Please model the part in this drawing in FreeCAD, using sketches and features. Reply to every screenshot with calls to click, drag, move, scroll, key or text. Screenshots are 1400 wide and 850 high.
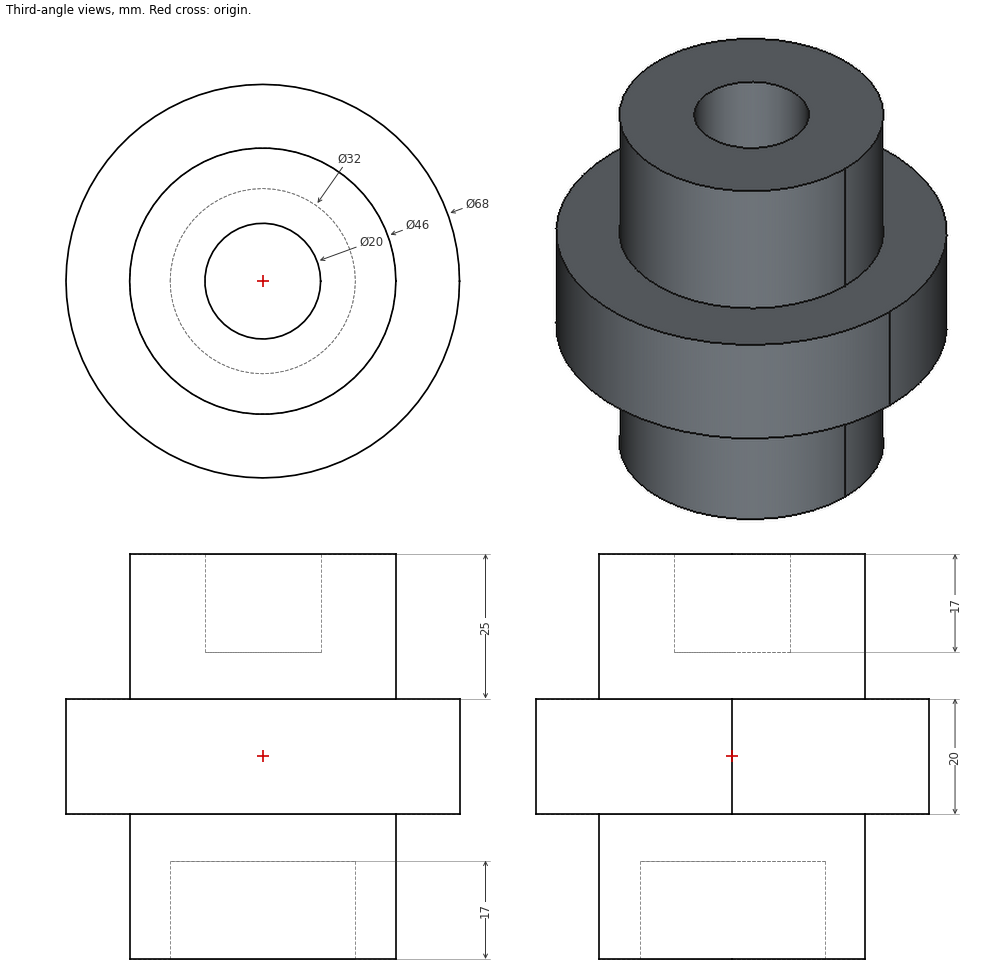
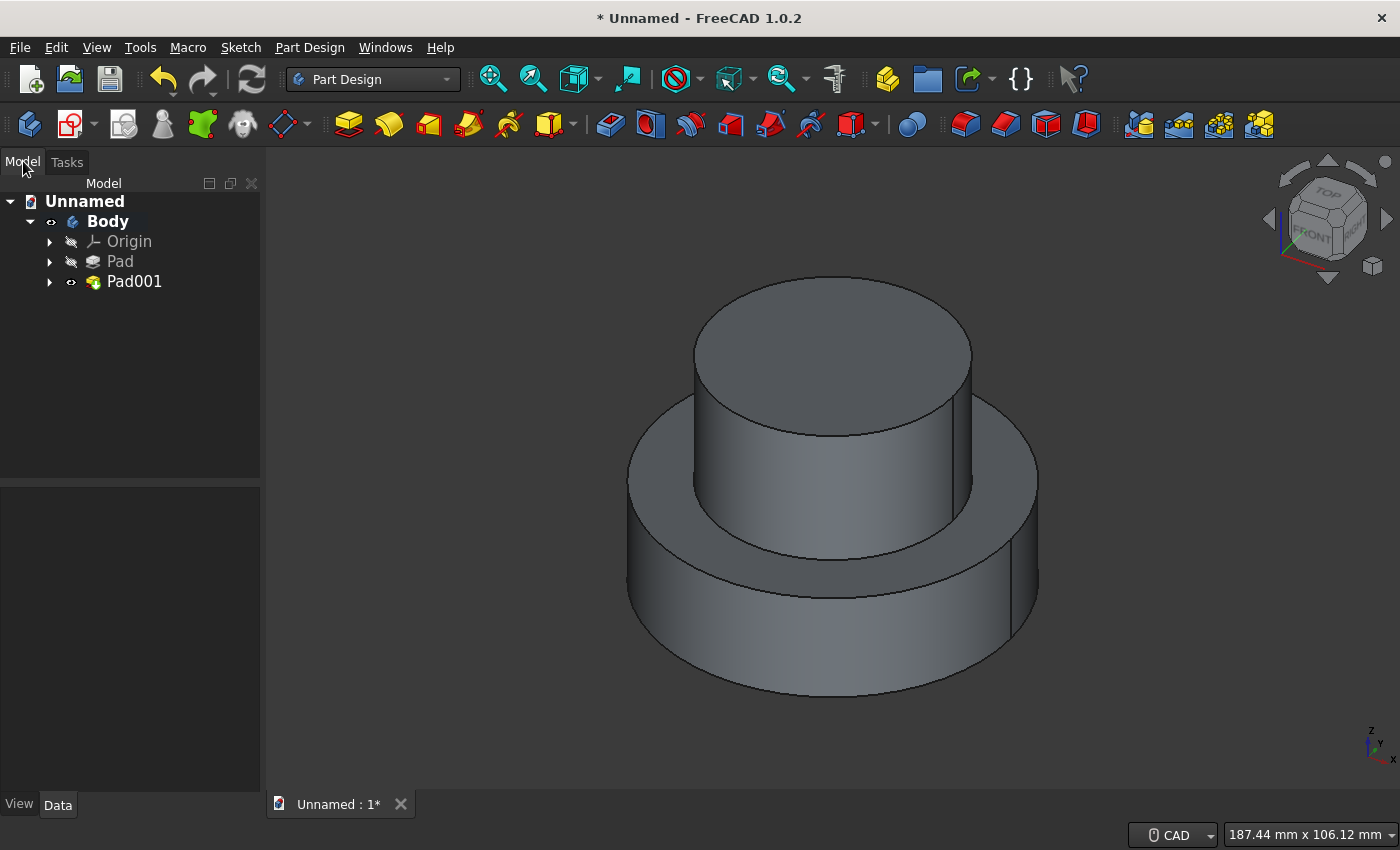
click(116, 282)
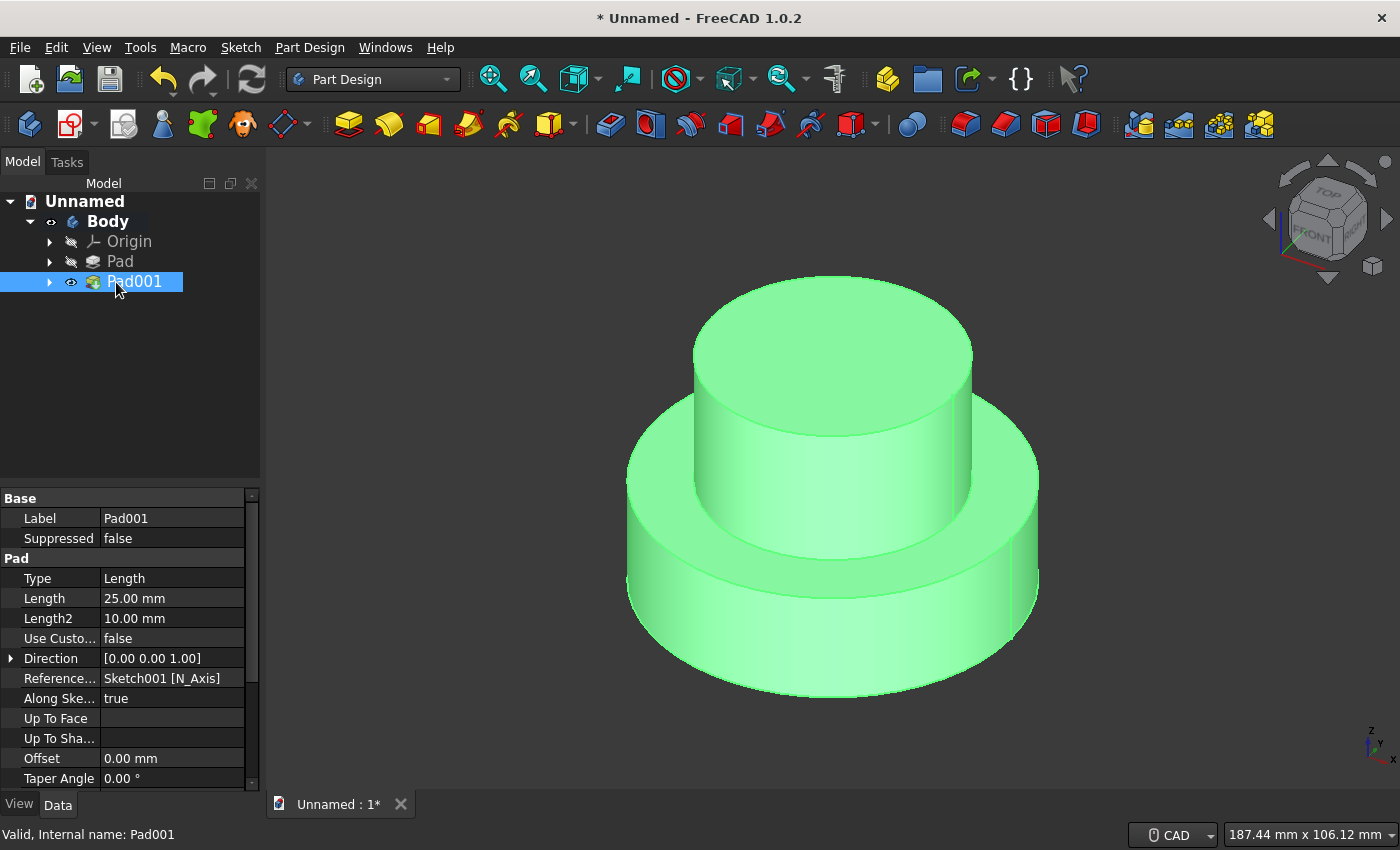
click(1140, 124)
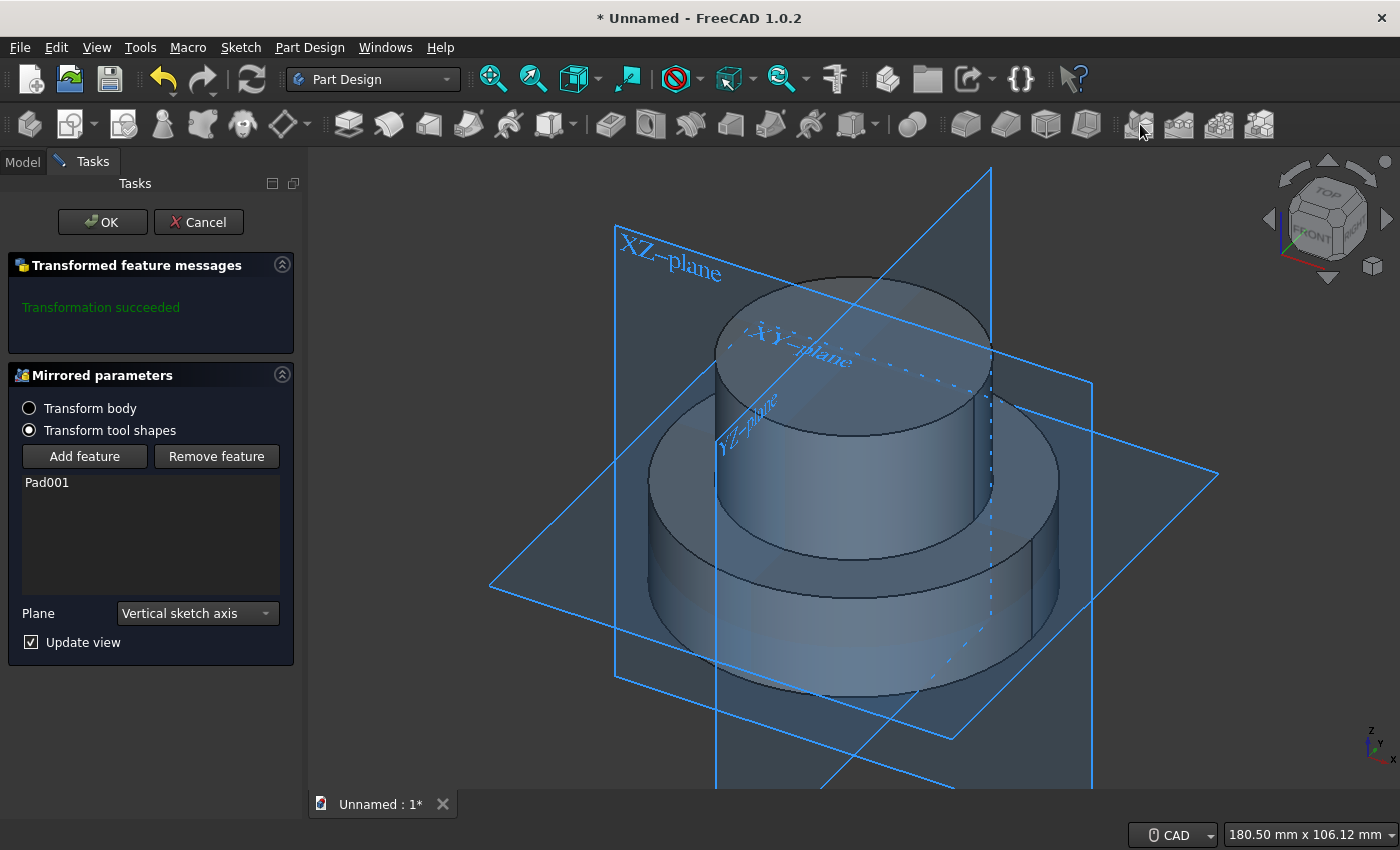
click(198, 614)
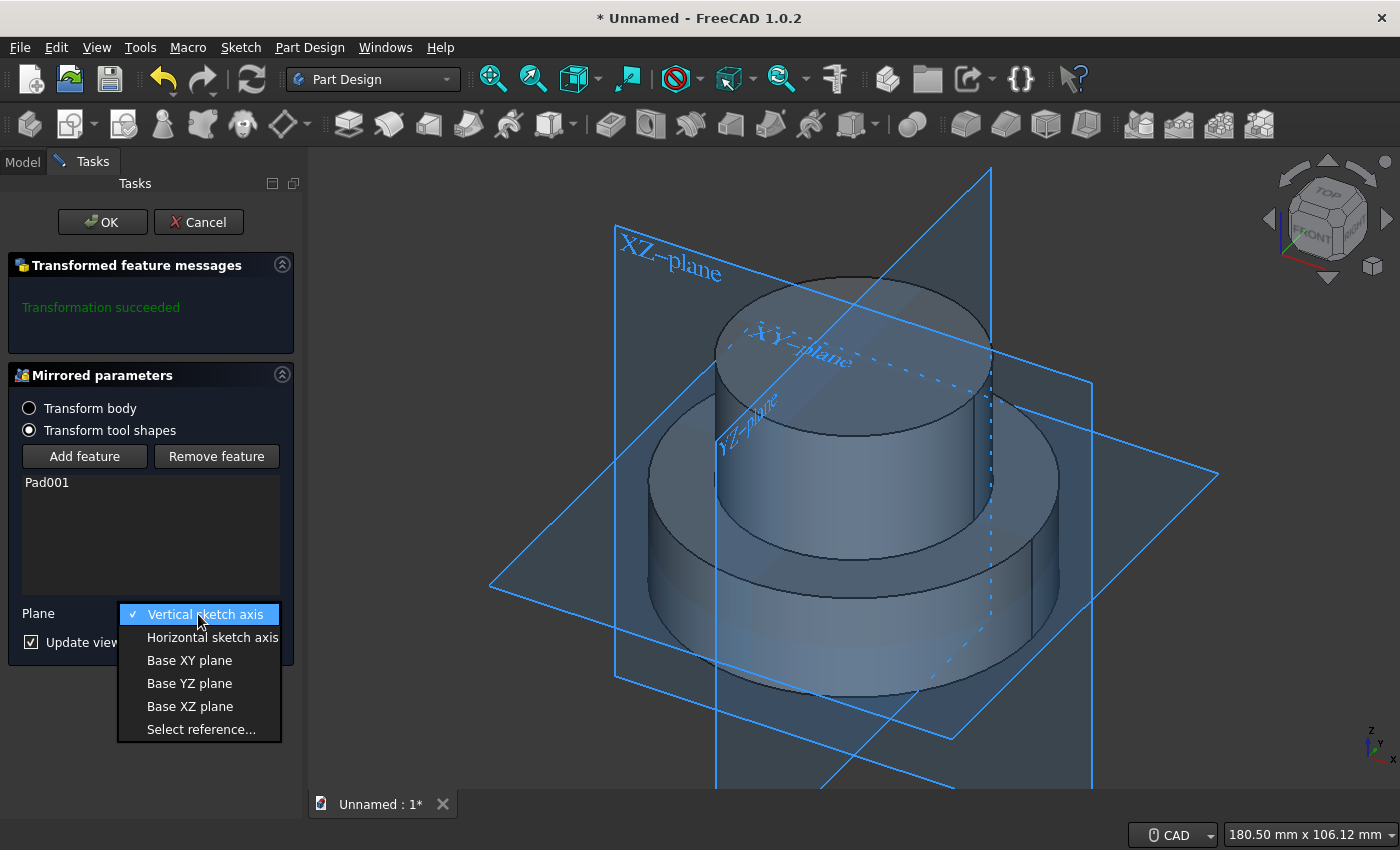
click(198, 660)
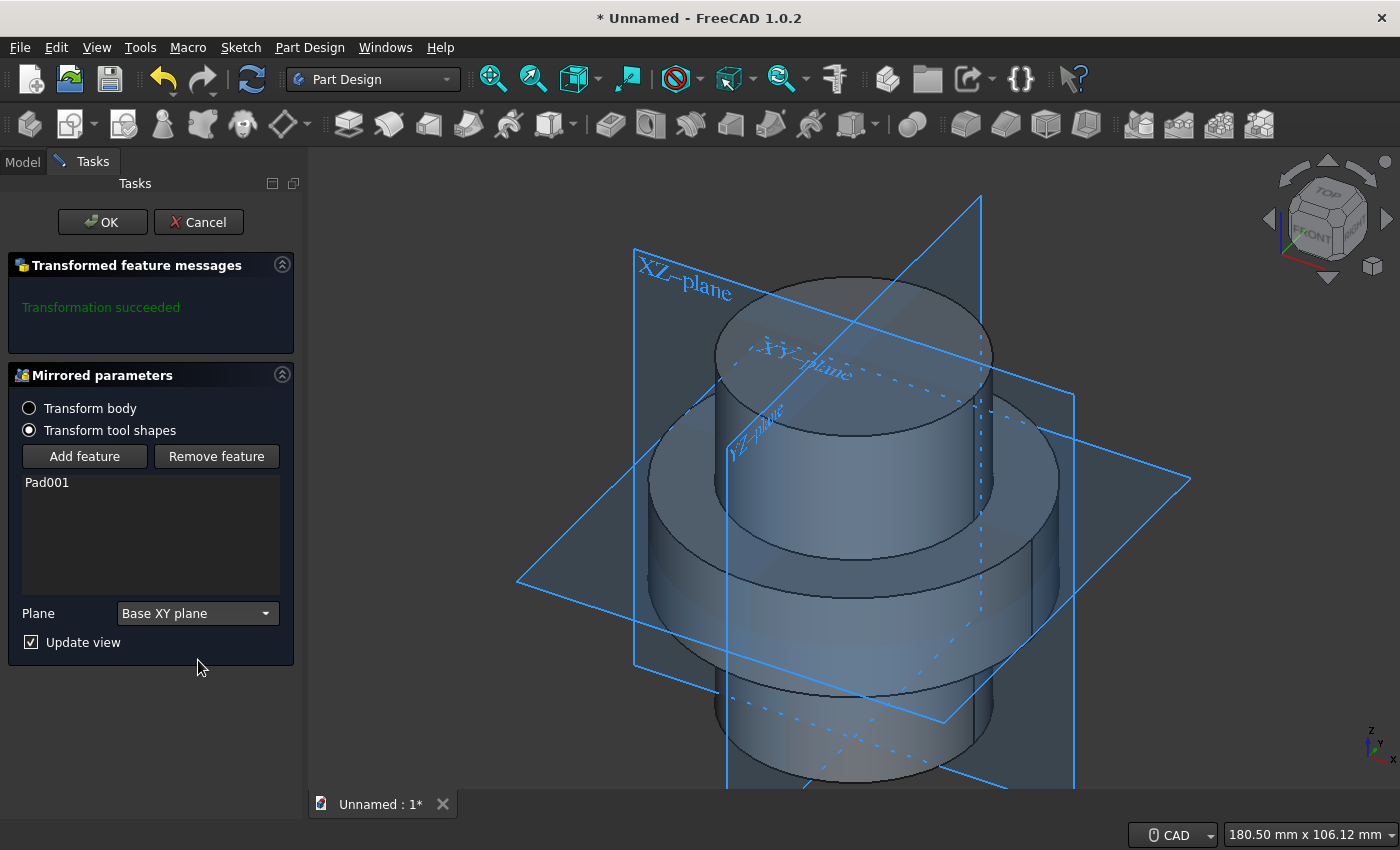
click(103, 222)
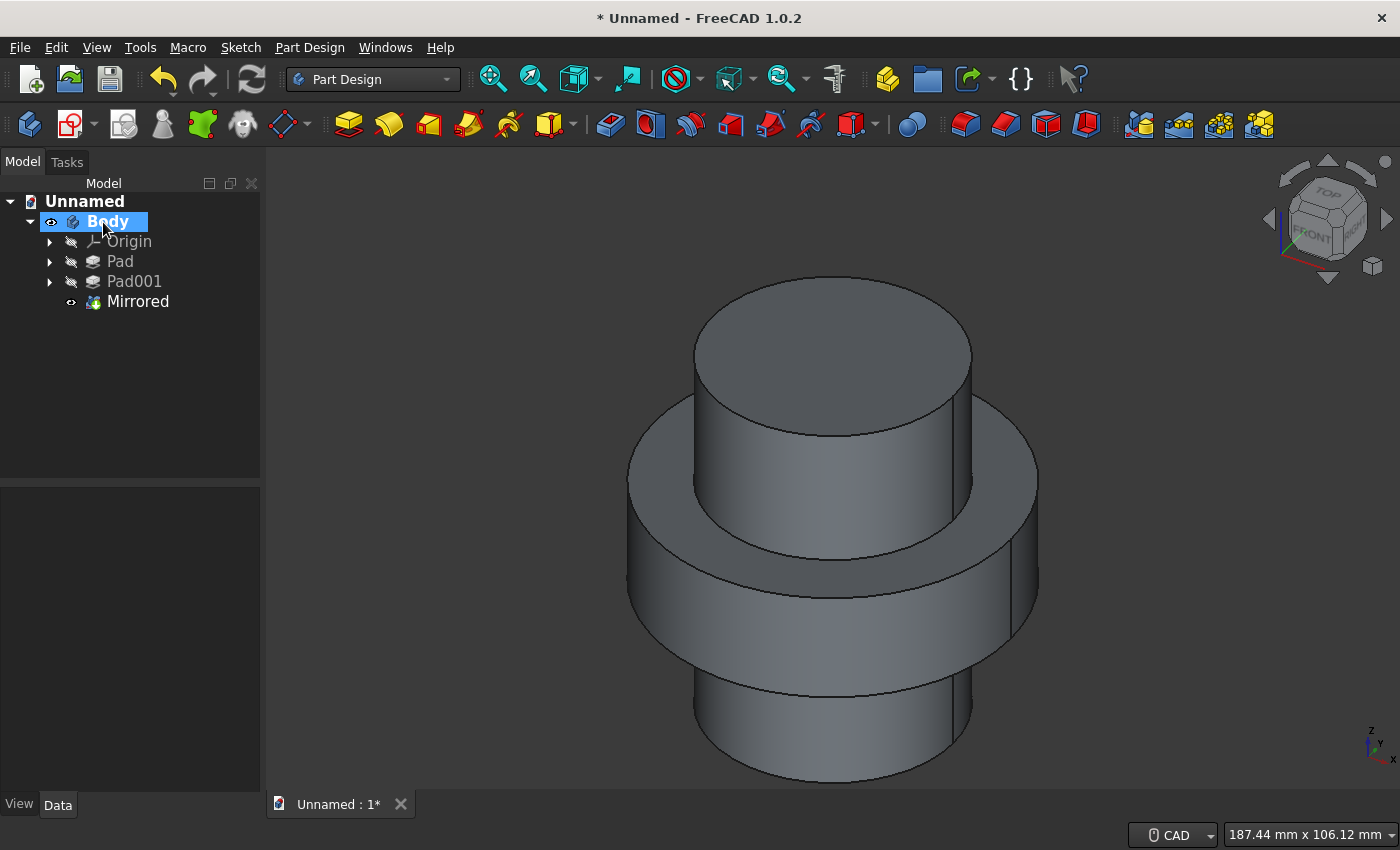
click(494, 80)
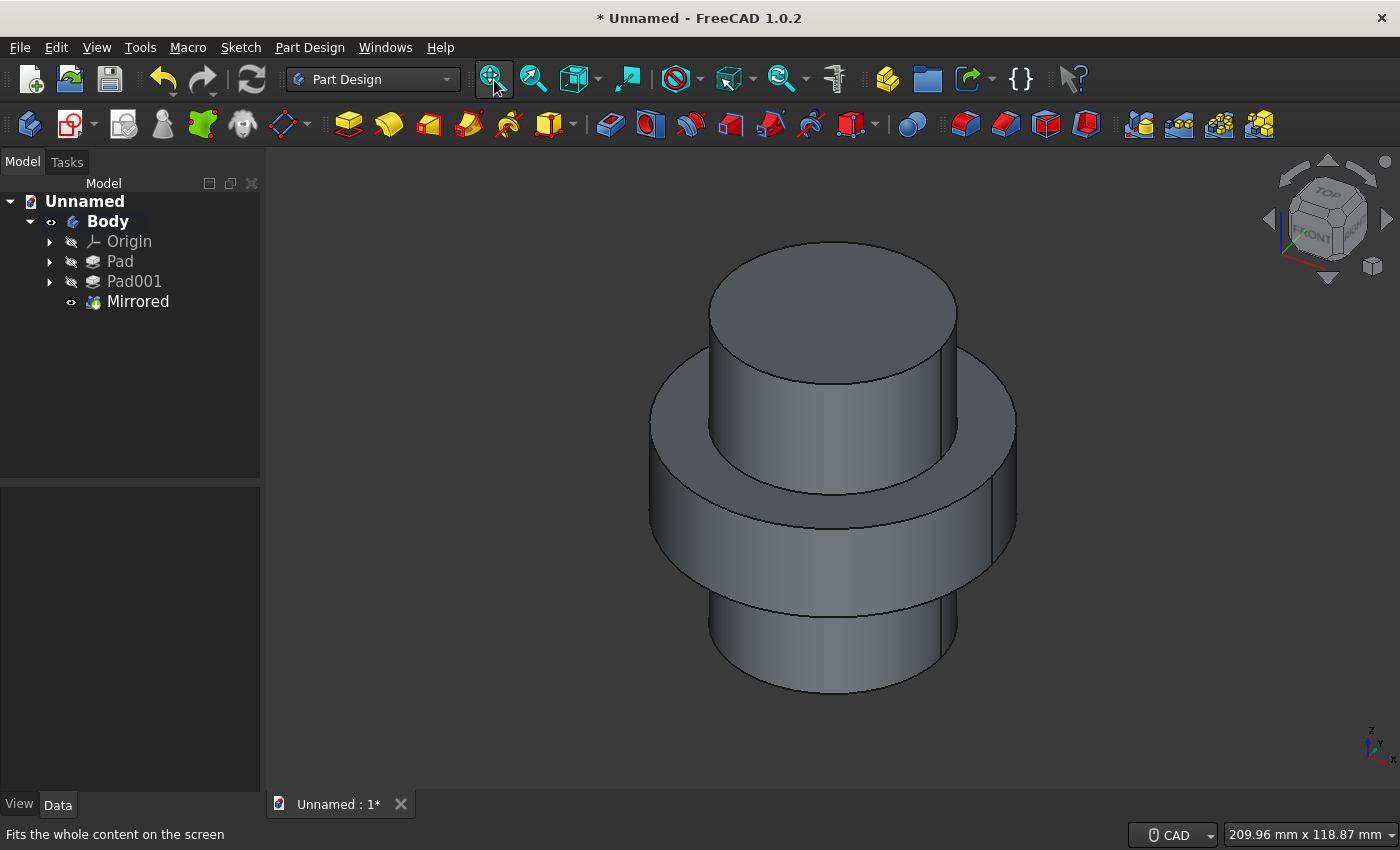
click(833, 312)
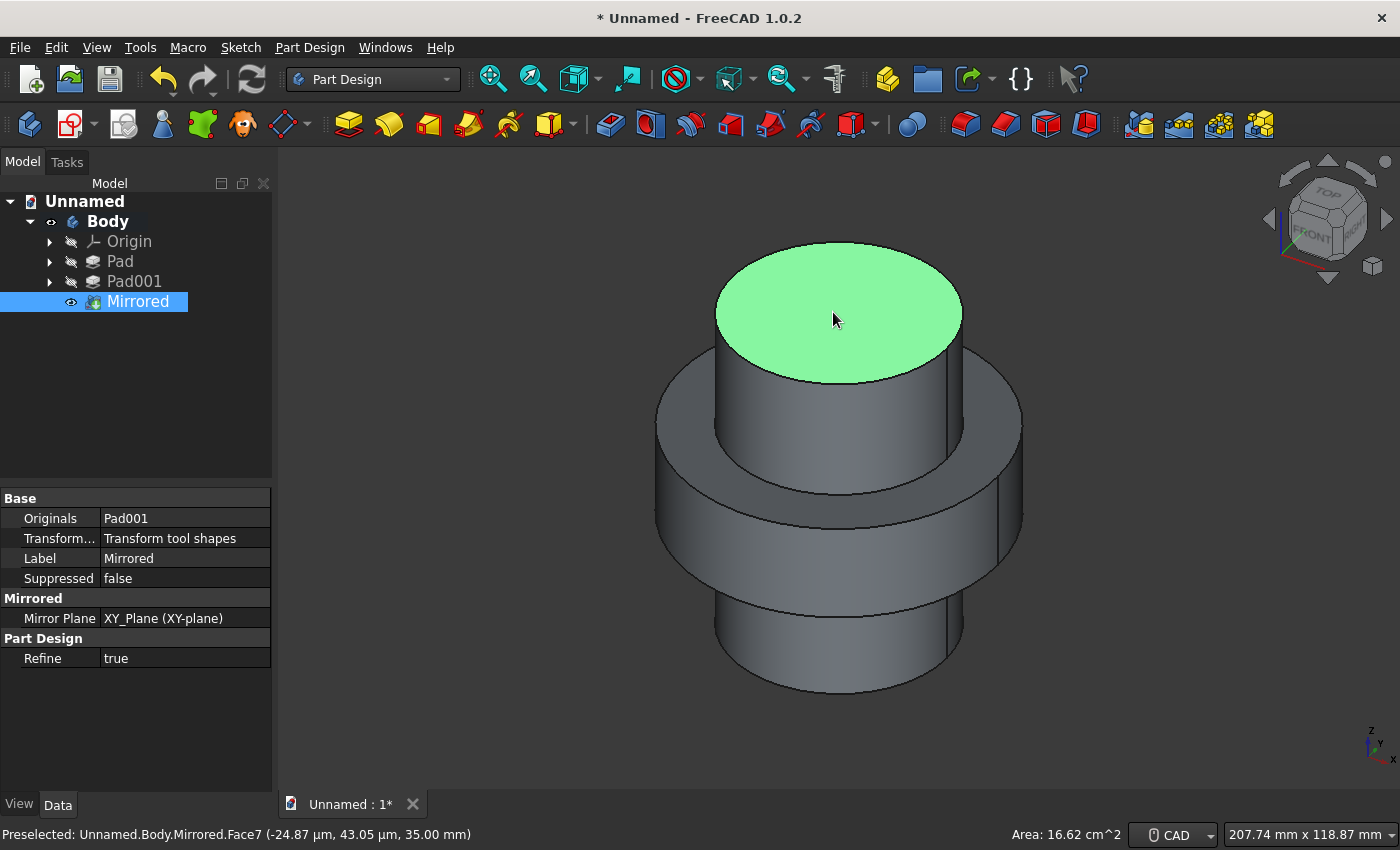
click(70, 124)